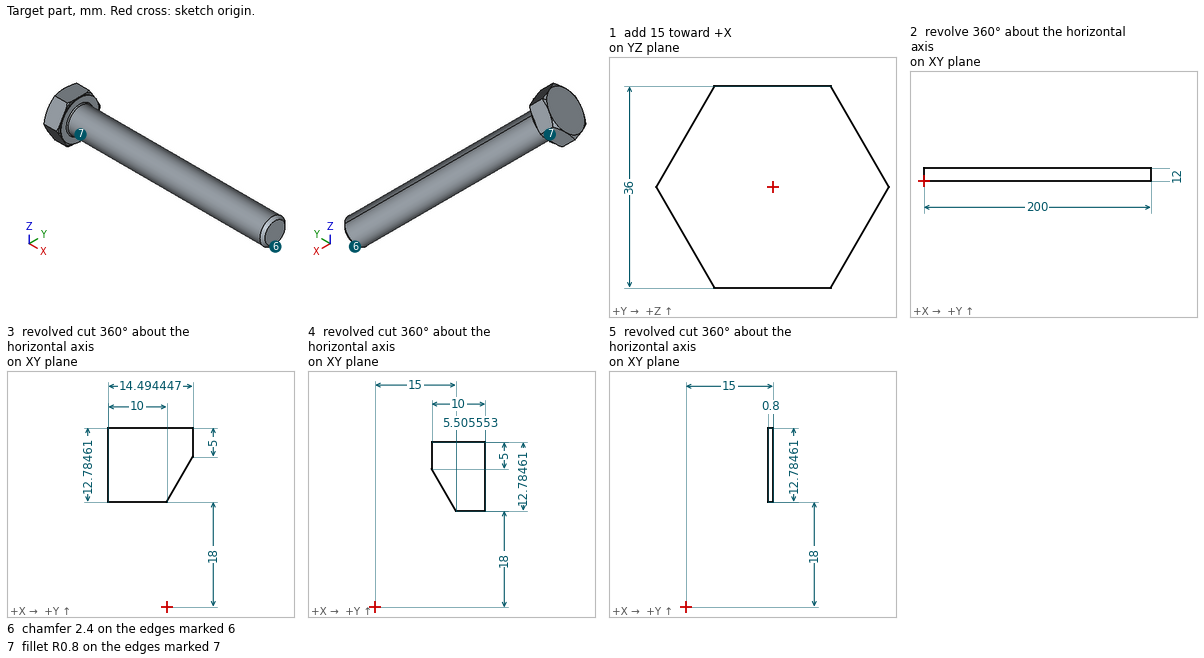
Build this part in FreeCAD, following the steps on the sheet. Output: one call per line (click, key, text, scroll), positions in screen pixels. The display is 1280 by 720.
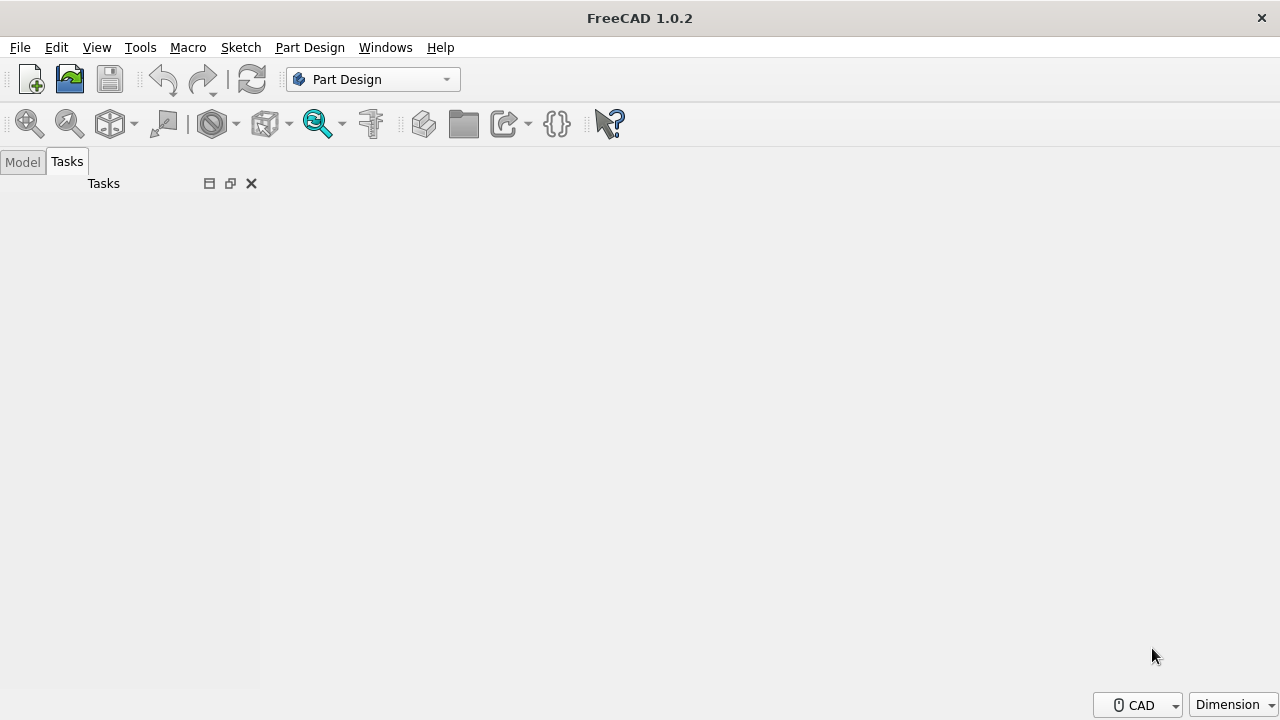
click(836, 80)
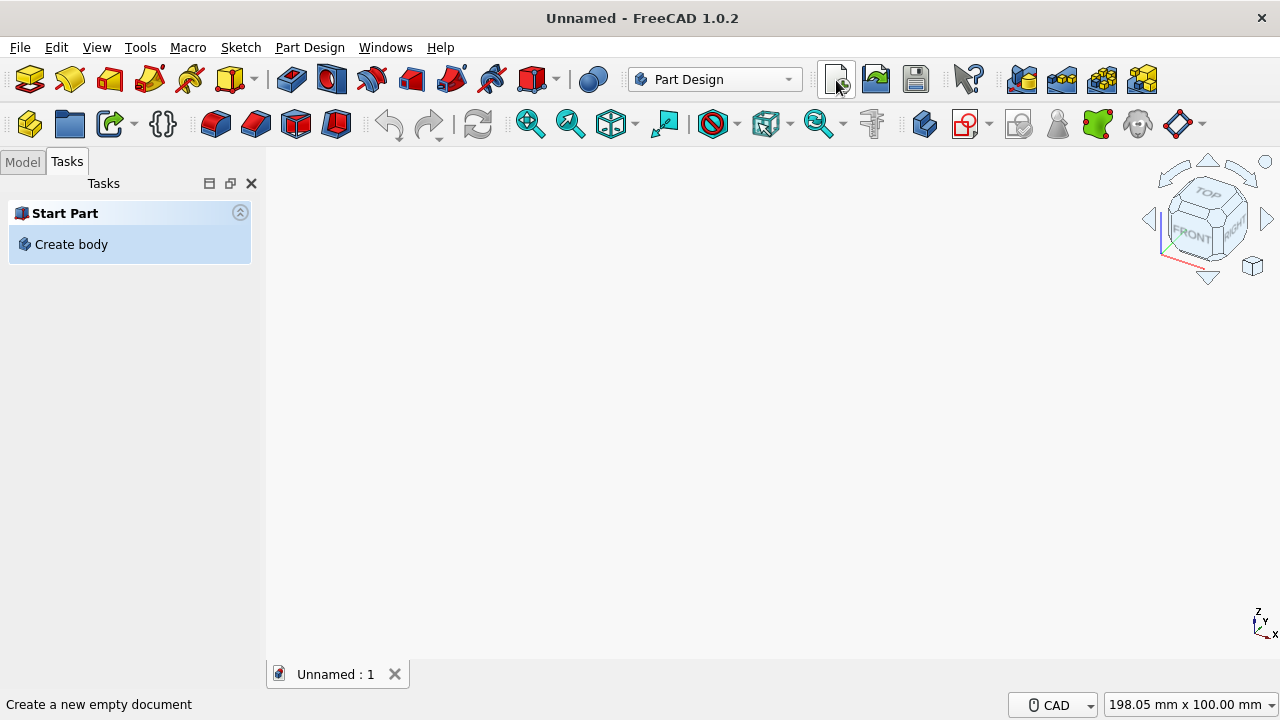
click(966, 124)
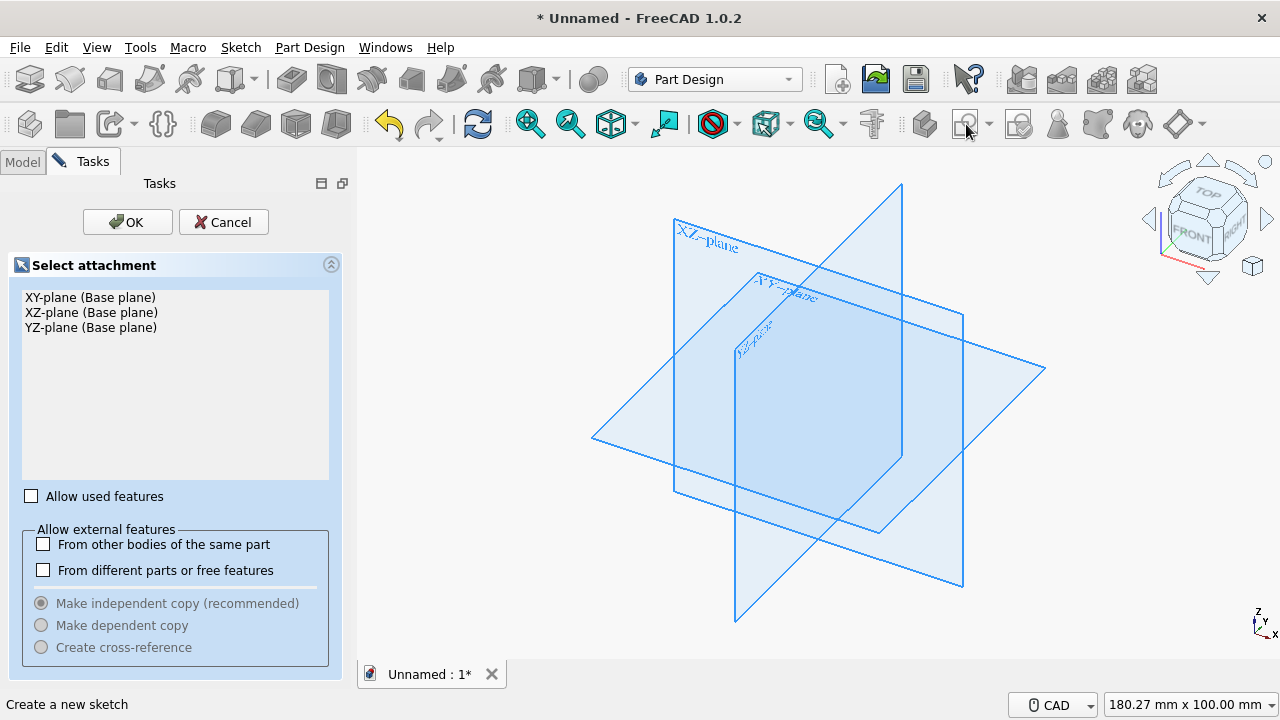
click(82, 328)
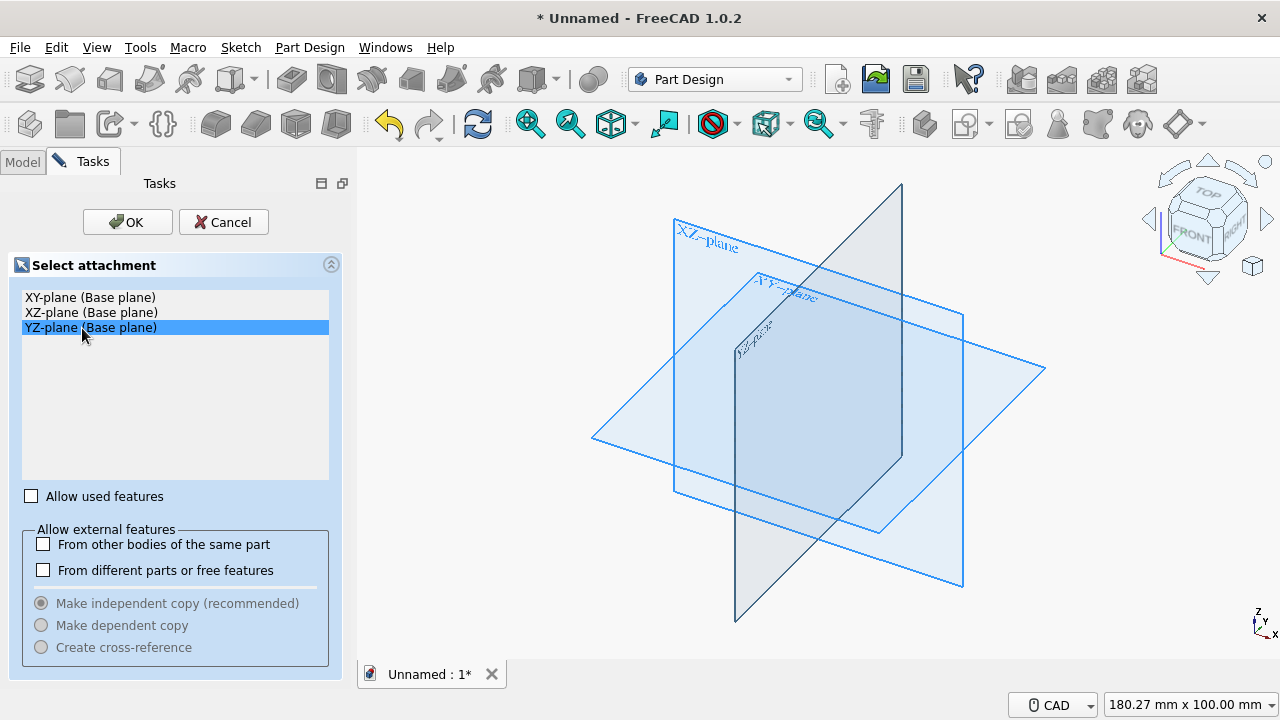
click(128, 222)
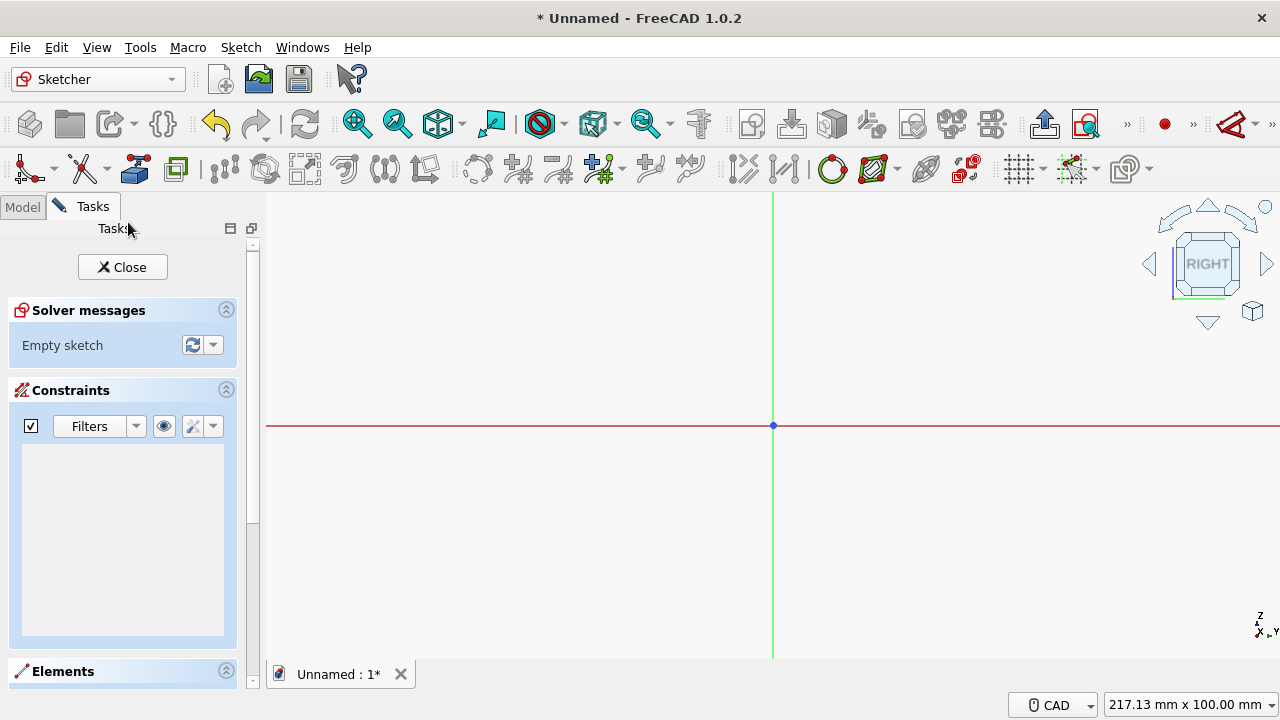
scroll(856, 426, up, 3)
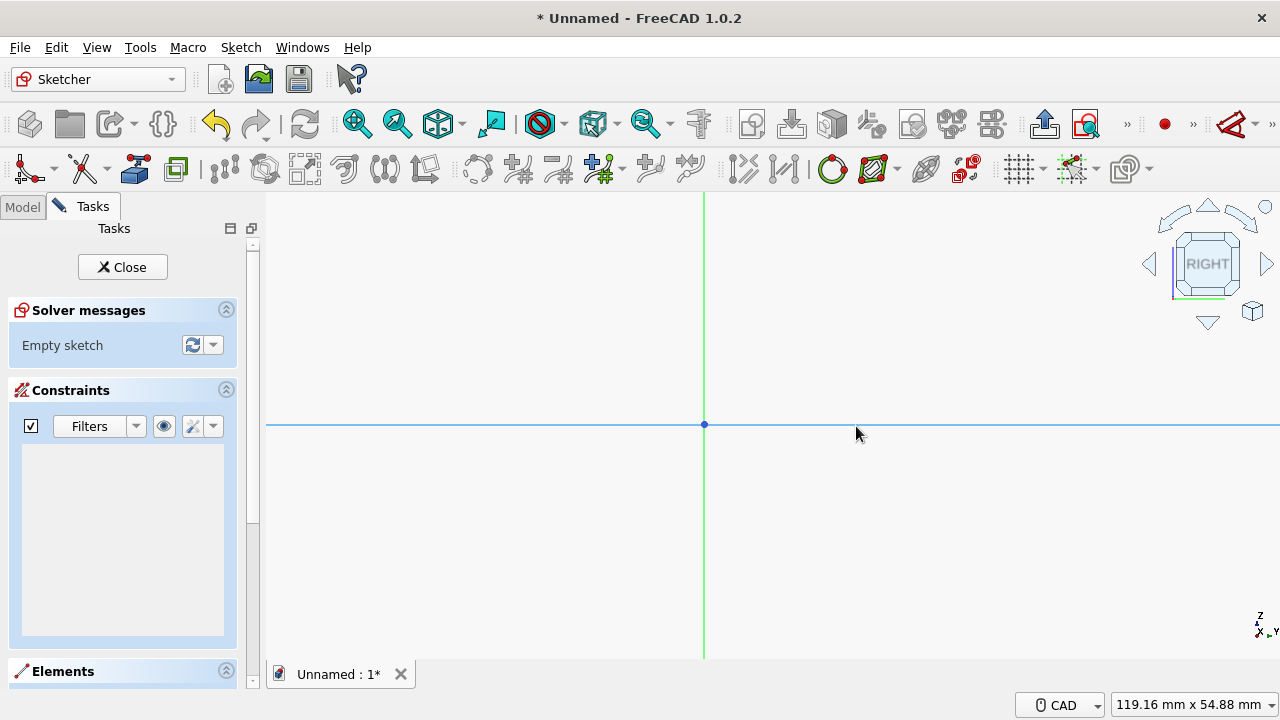
key(g)
key(p)
key(6)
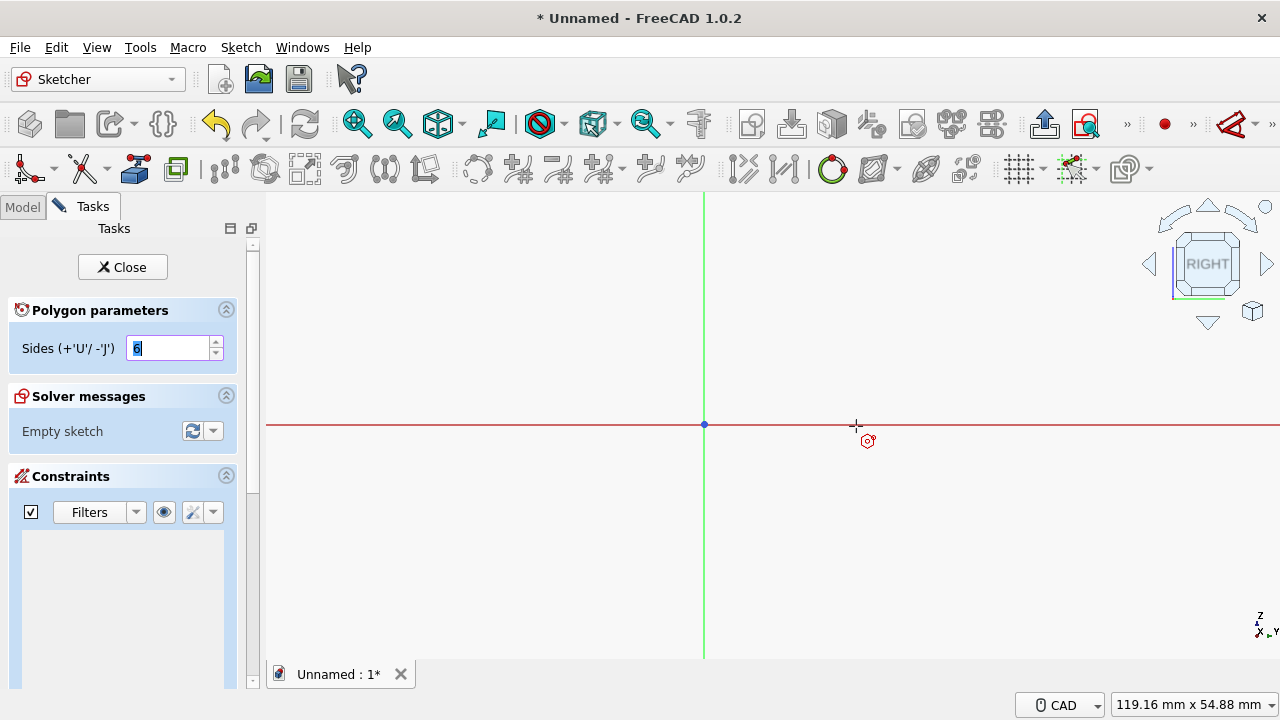
click(704, 425)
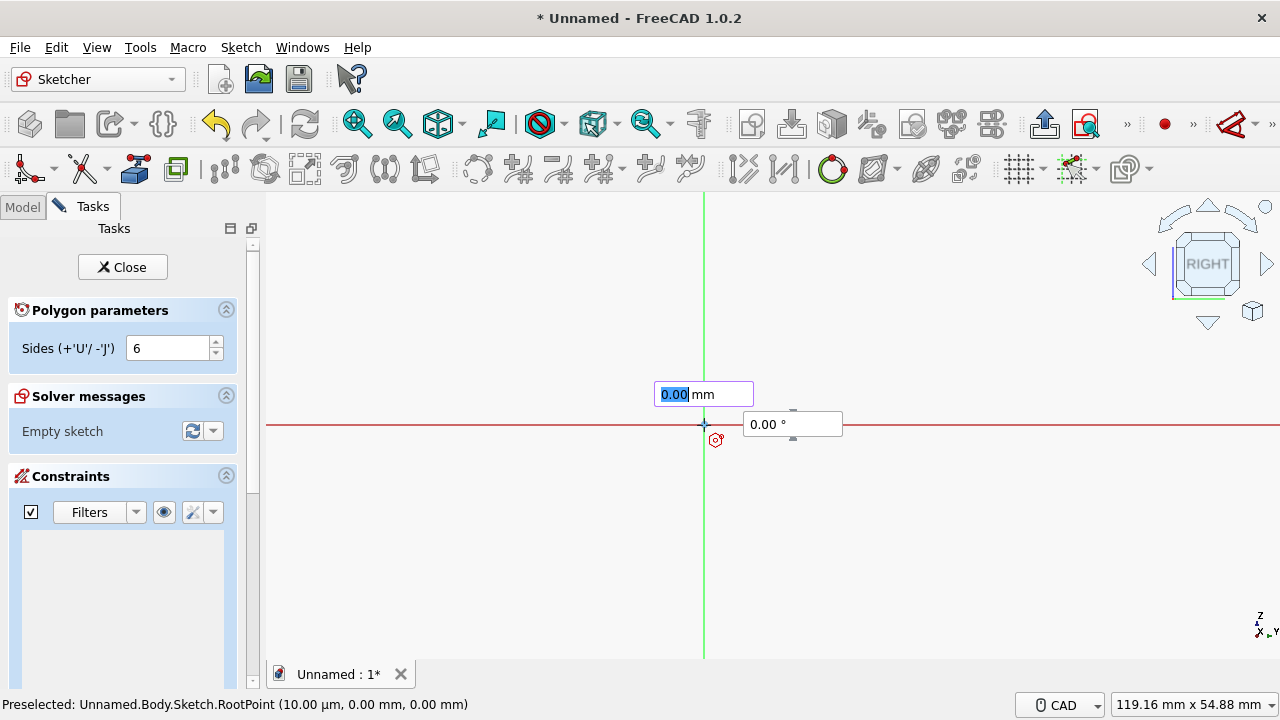
click(881, 425)
right_click(881, 425)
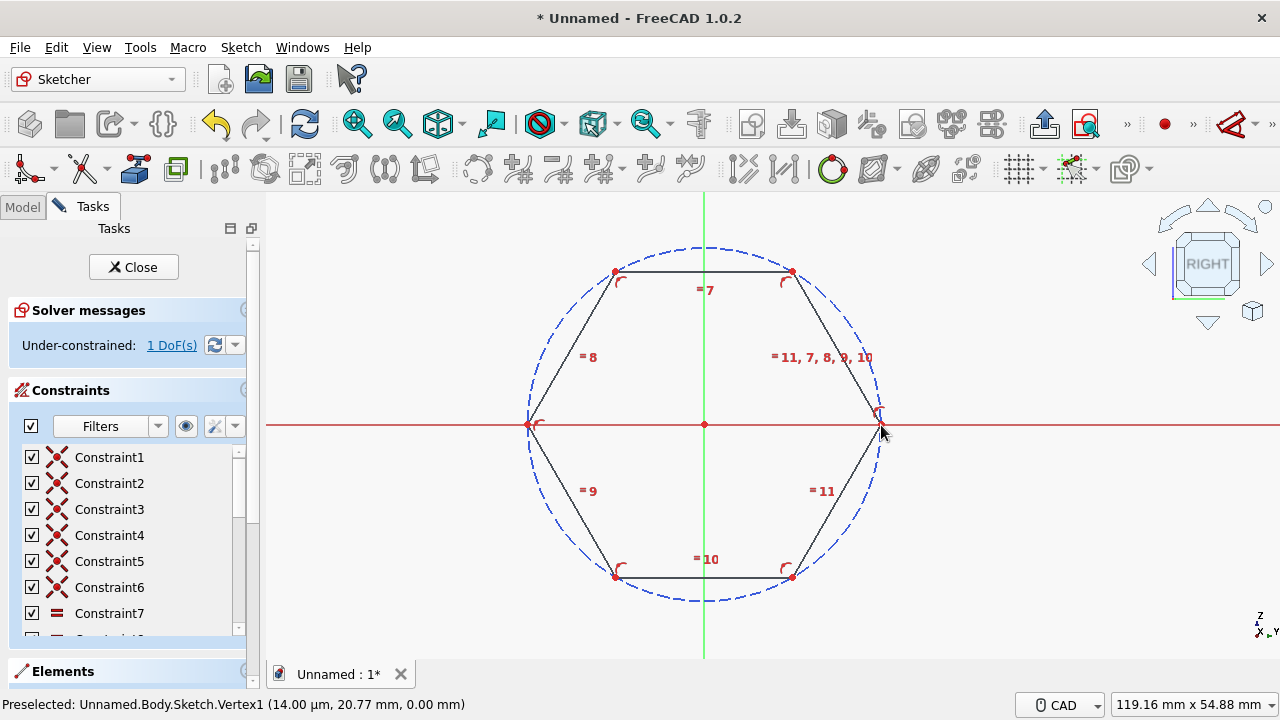
click(1232, 124)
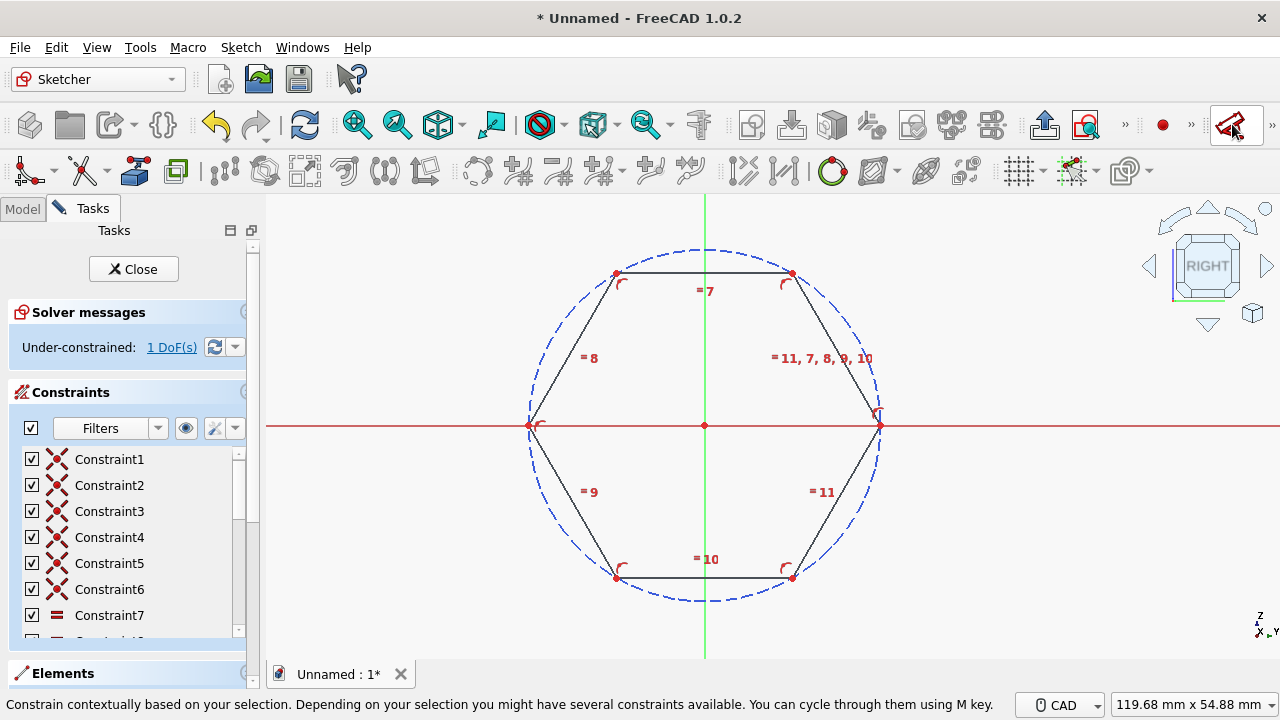
click(617, 578)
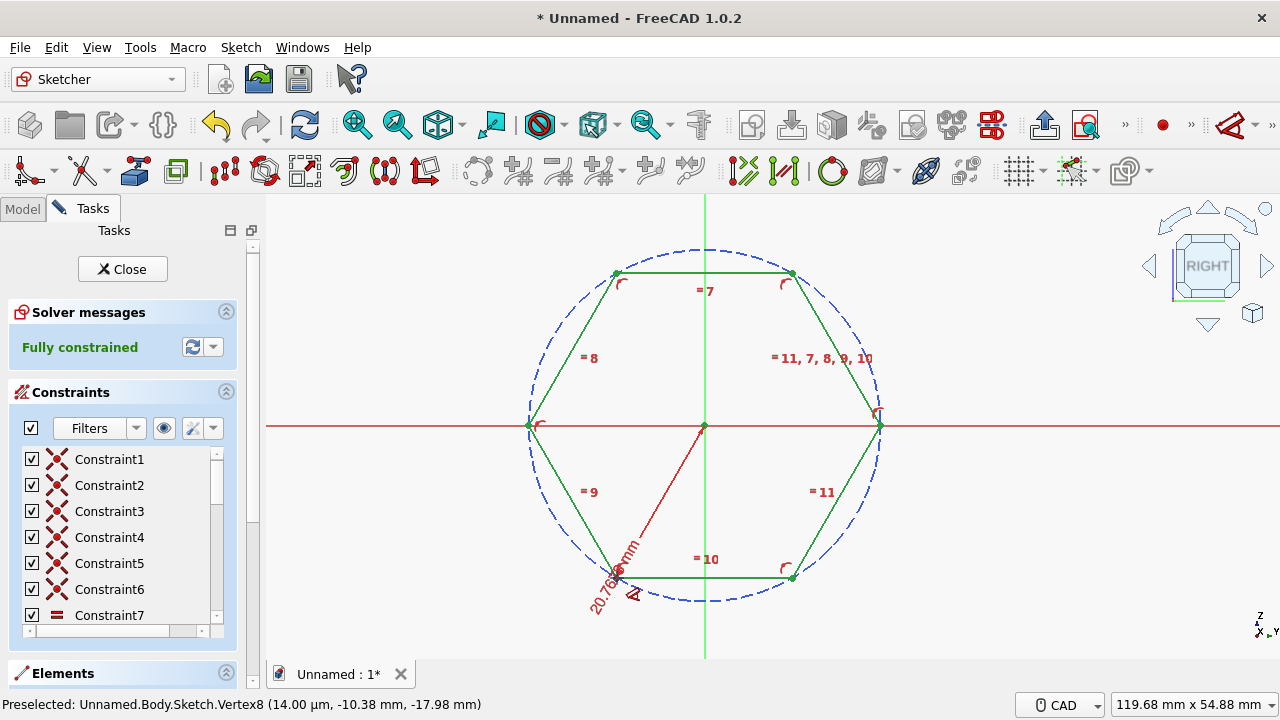
click(793, 273)
click(875, 319)